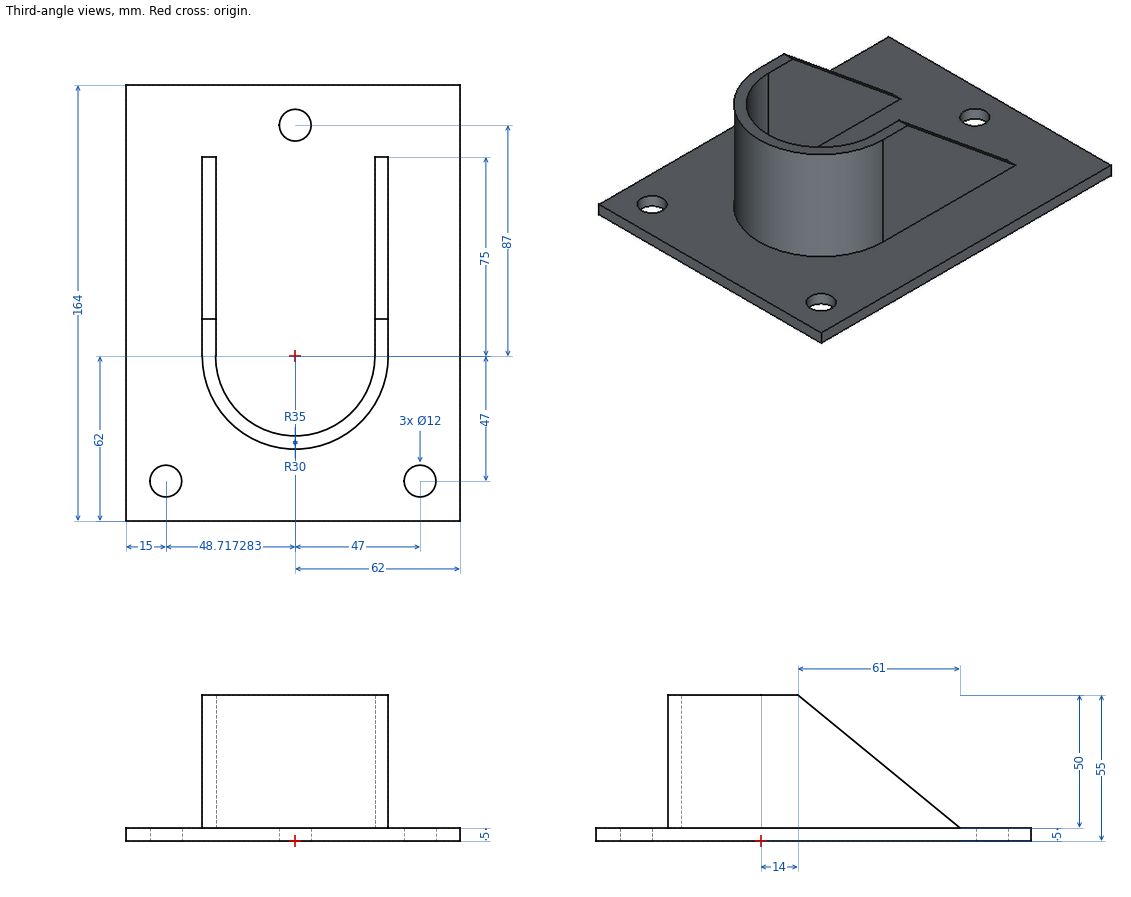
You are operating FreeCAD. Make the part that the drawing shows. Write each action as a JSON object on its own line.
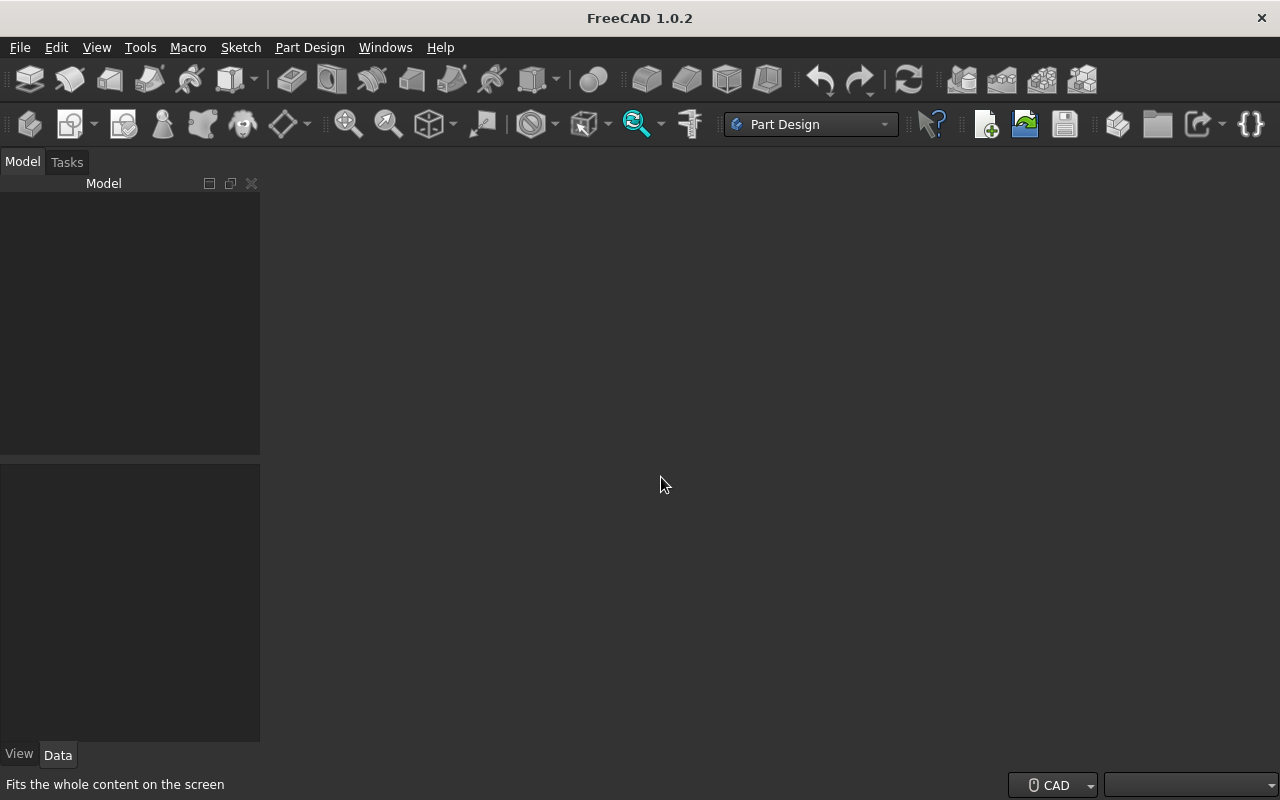
{"action": "left_click", "coordinate": [986, 124]}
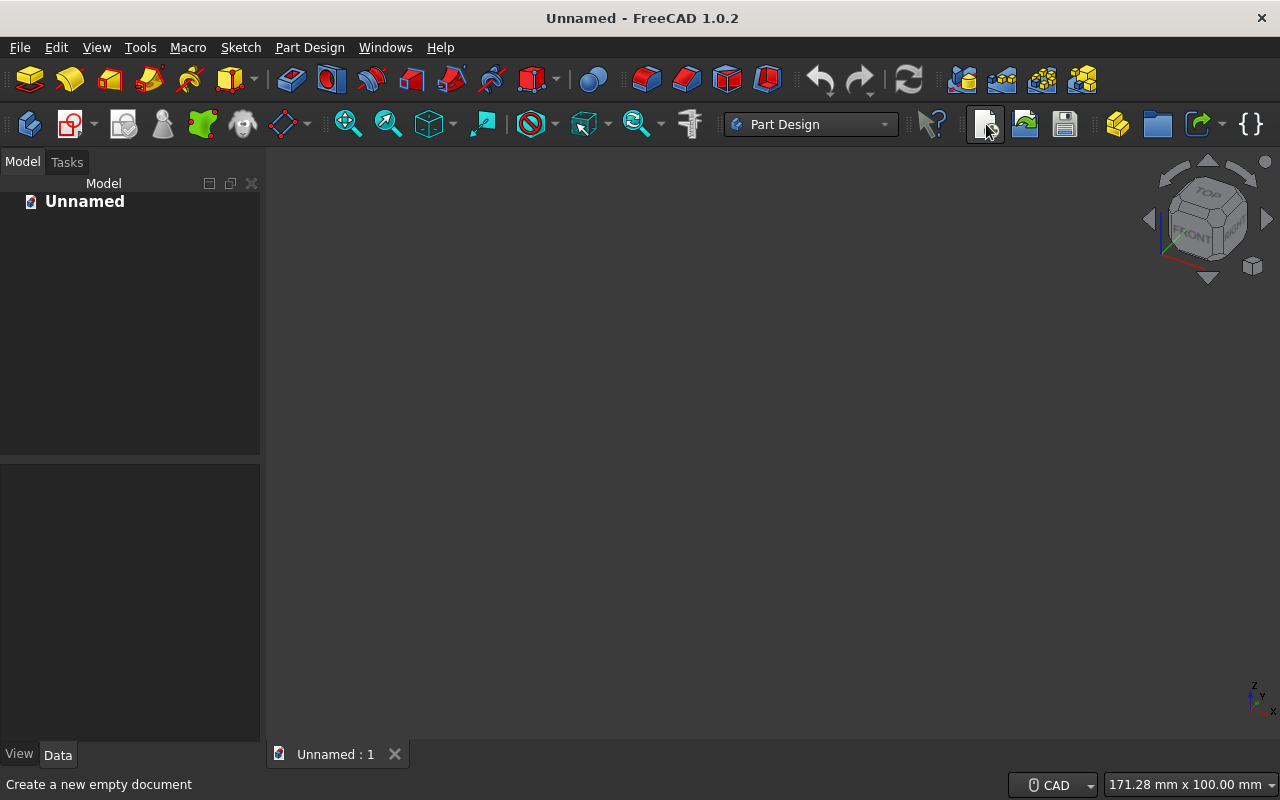
{"action": "left_click", "coordinate": [70, 124]}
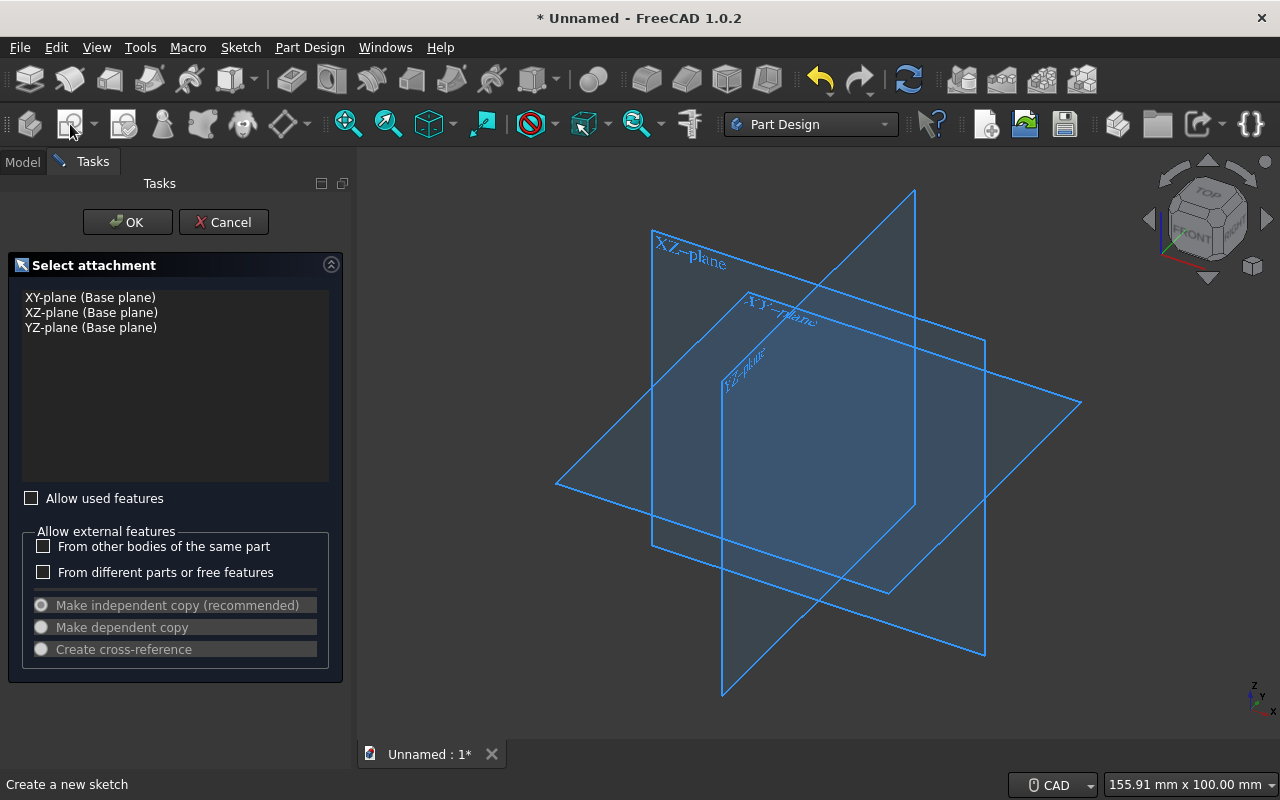
{"action": "left_click", "coordinate": [82, 298]}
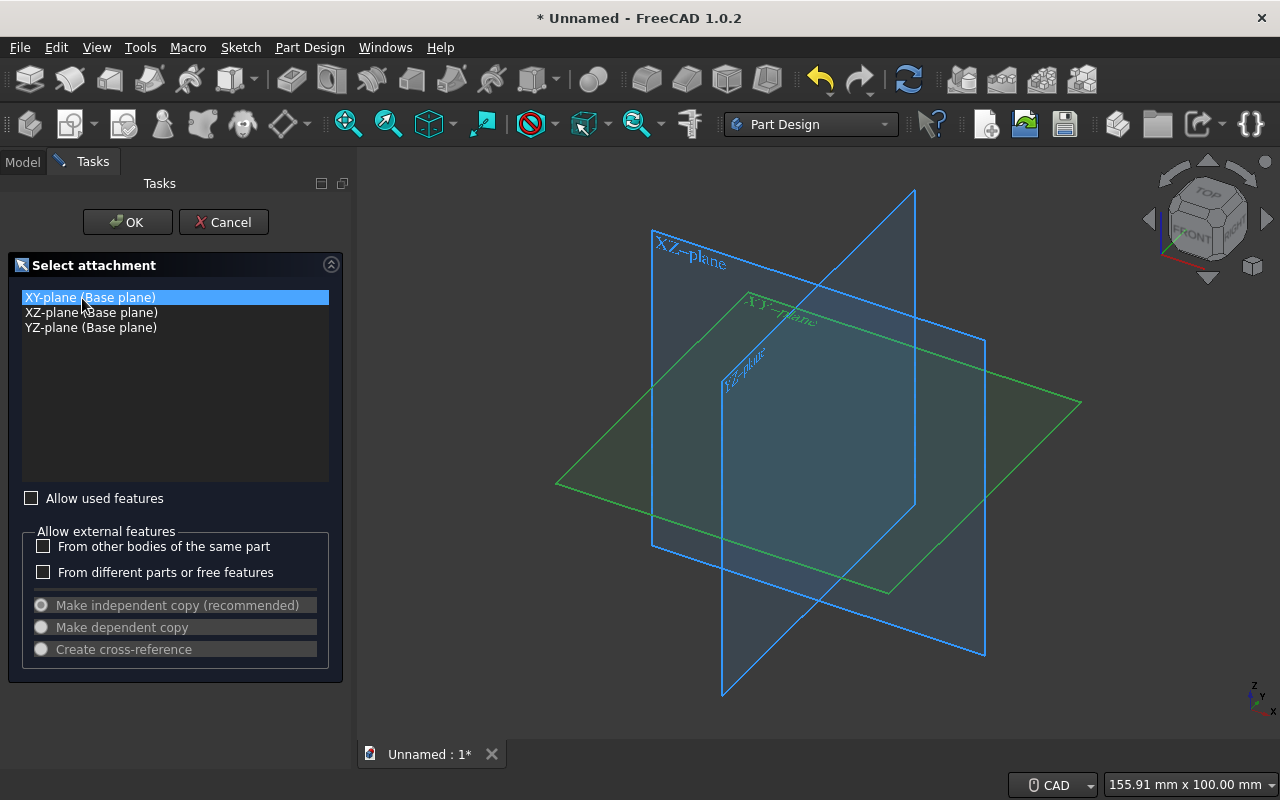
{"action": "left_click", "coordinate": [128, 222]}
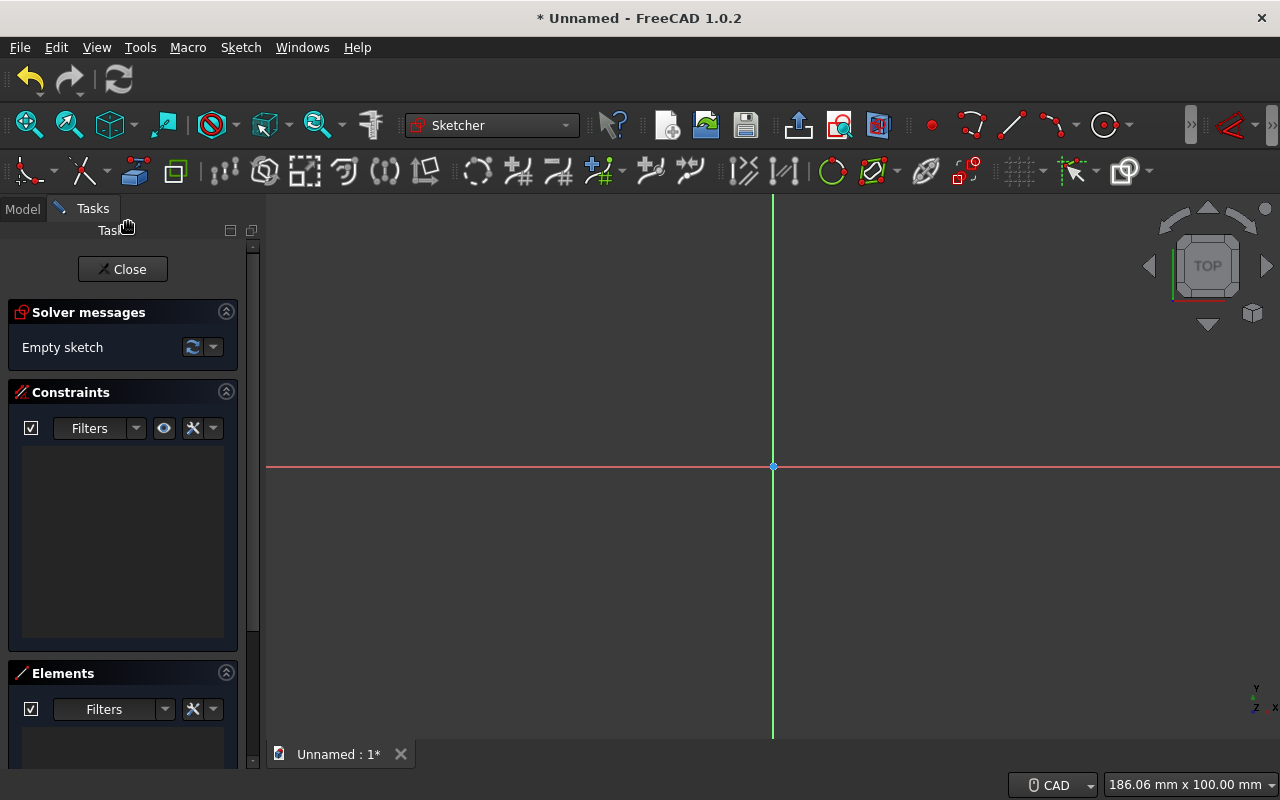
{"action": "scroll", "coordinate": [621, 599], "scroll_direction": "down", "scroll_amount": 3}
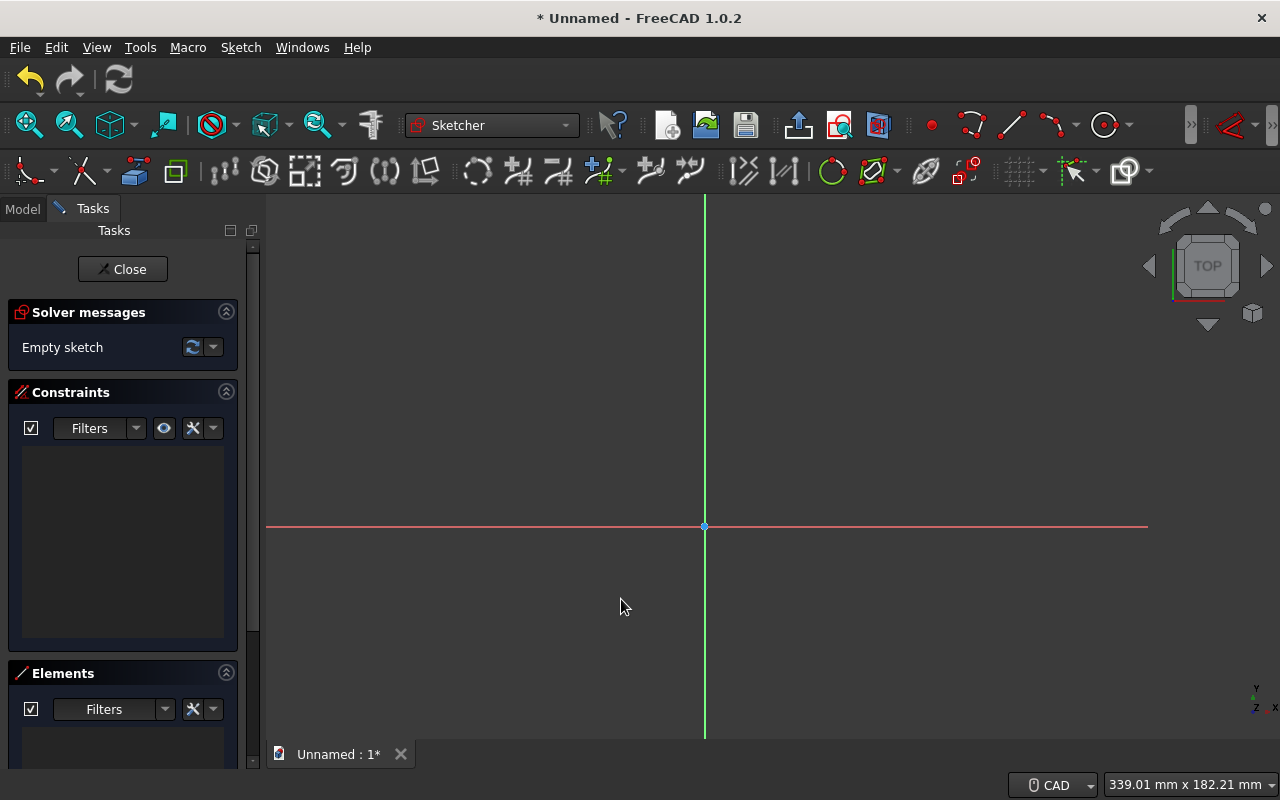
{"action": "left_click", "coordinate": [972, 126]}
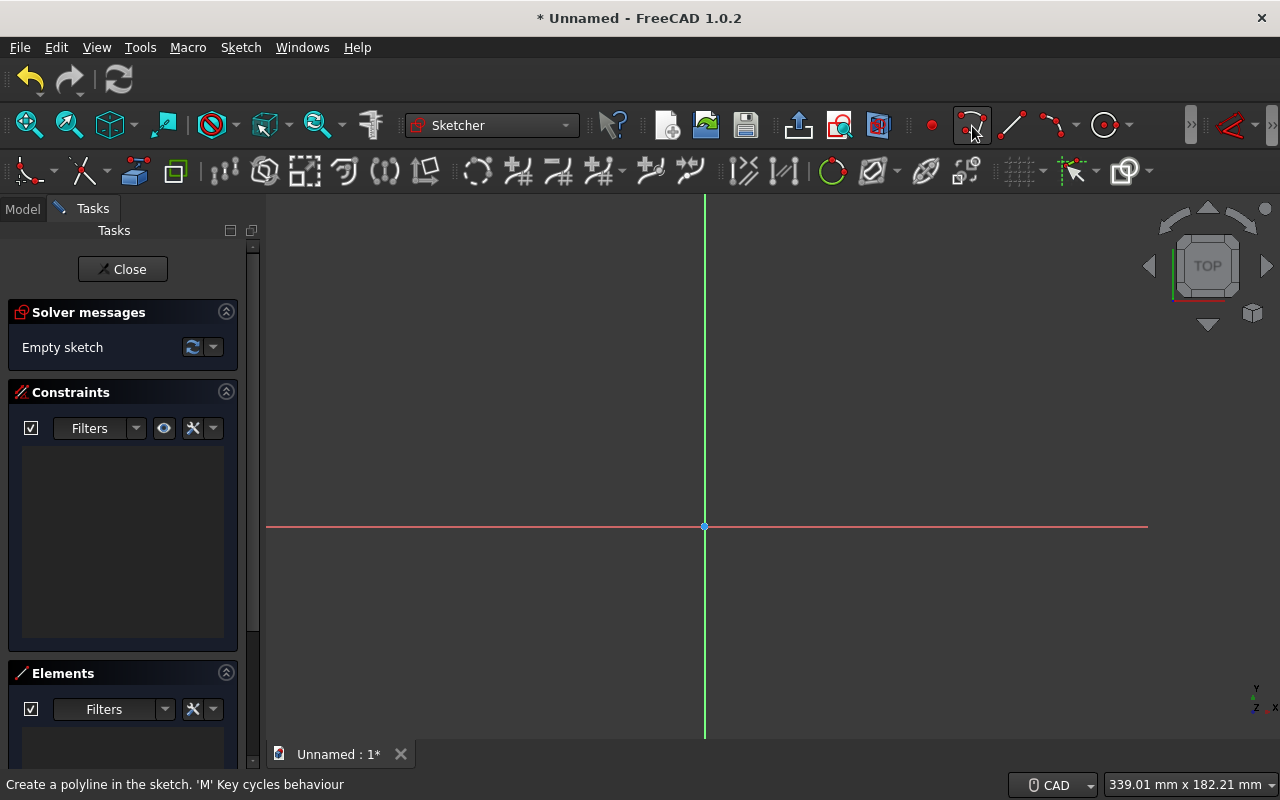
{"action": "left_click", "coordinate": [809, 527]}
{"action": "left_click", "coordinate": [809, 302]}
{"action": "left_click", "coordinate": [794, 302]}
{"action": "left_click", "coordinate": [794, 527]}
{"action": "right_click", "coordinate": [794, 527]}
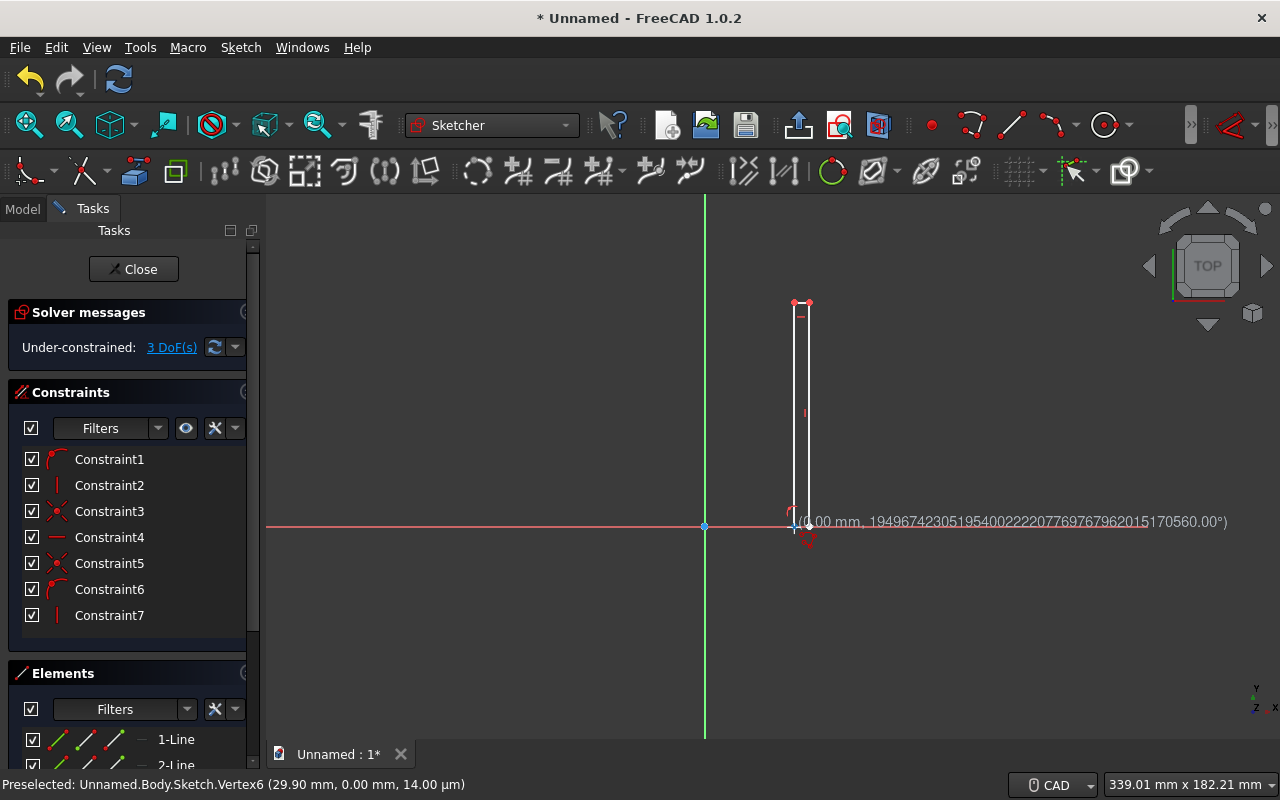
{"action": "left_click", "coordinate": [615, 527]}
{"action": "left_click", "coordinate": [615, 302]}
{"action": "left_click", "coordinate": [600, 302]}
{"action": "left_click", "coordinate": [600, 527]}
{"action": "right_click", "coordinate": [600, 527]}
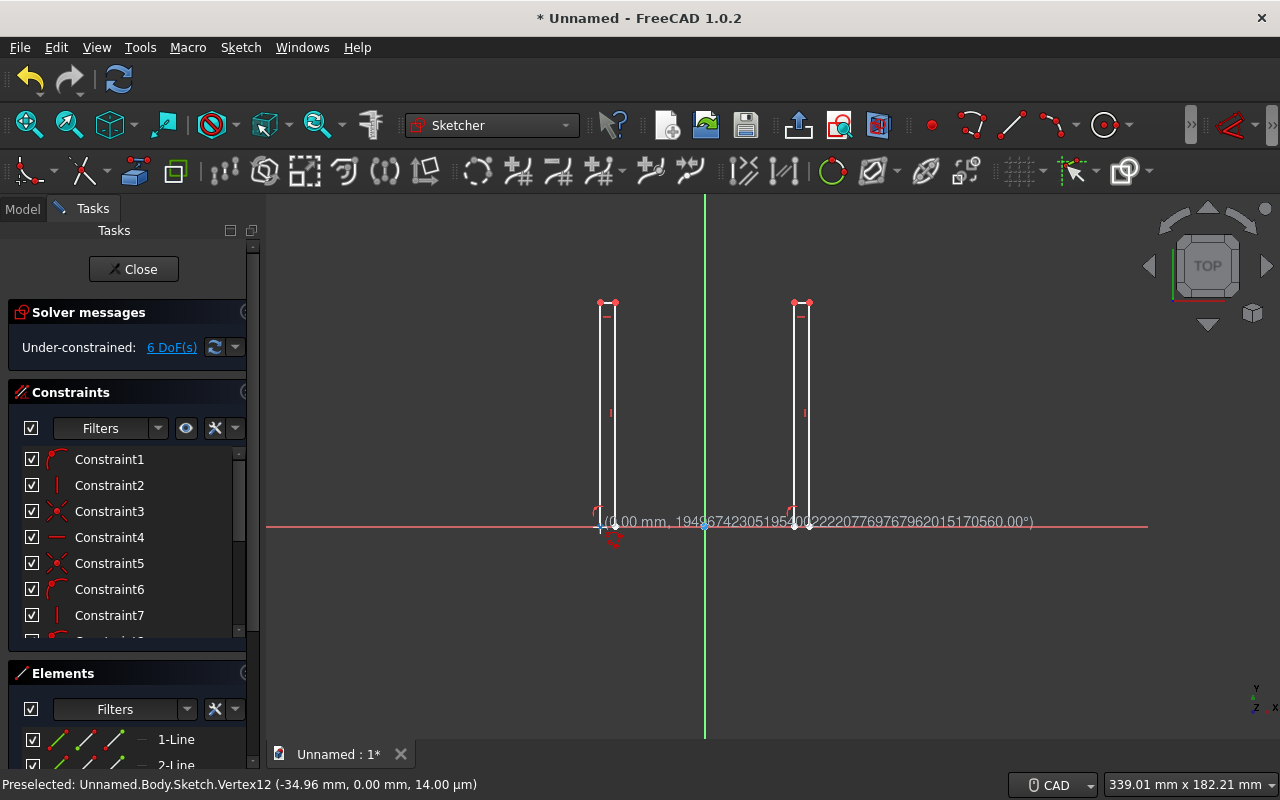
{"action": "left_click", "coordinate": [1052, 126]}